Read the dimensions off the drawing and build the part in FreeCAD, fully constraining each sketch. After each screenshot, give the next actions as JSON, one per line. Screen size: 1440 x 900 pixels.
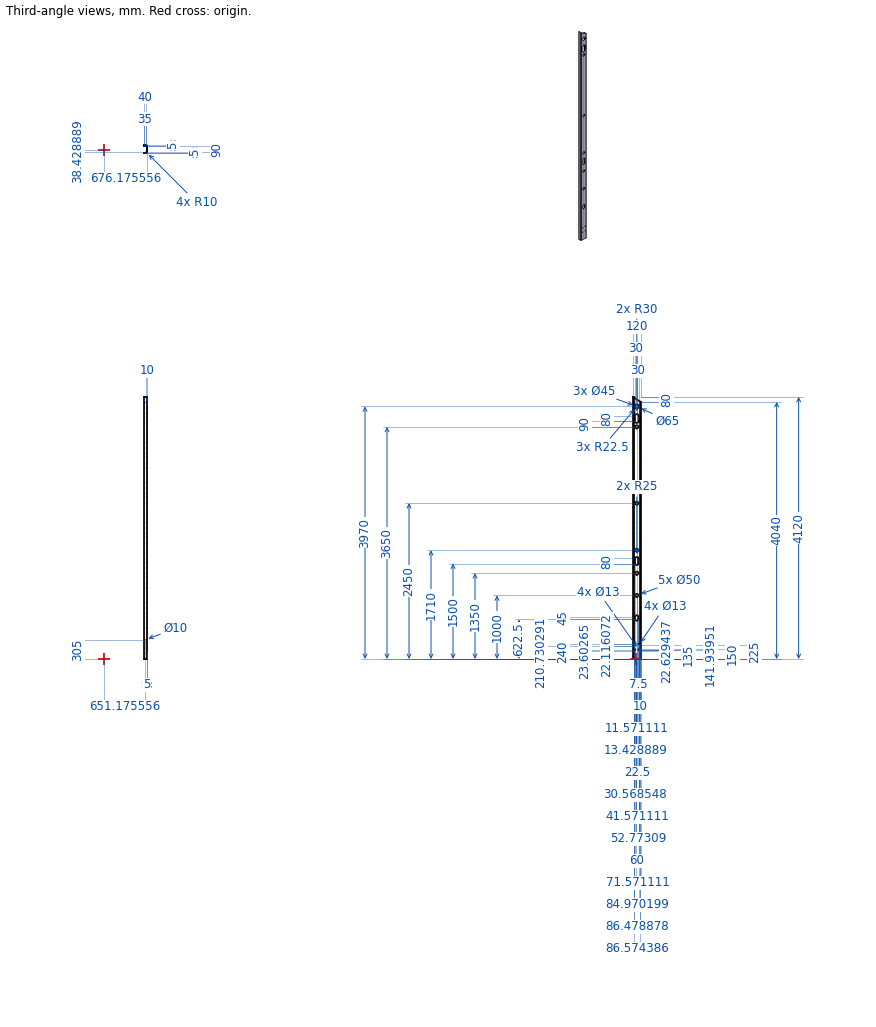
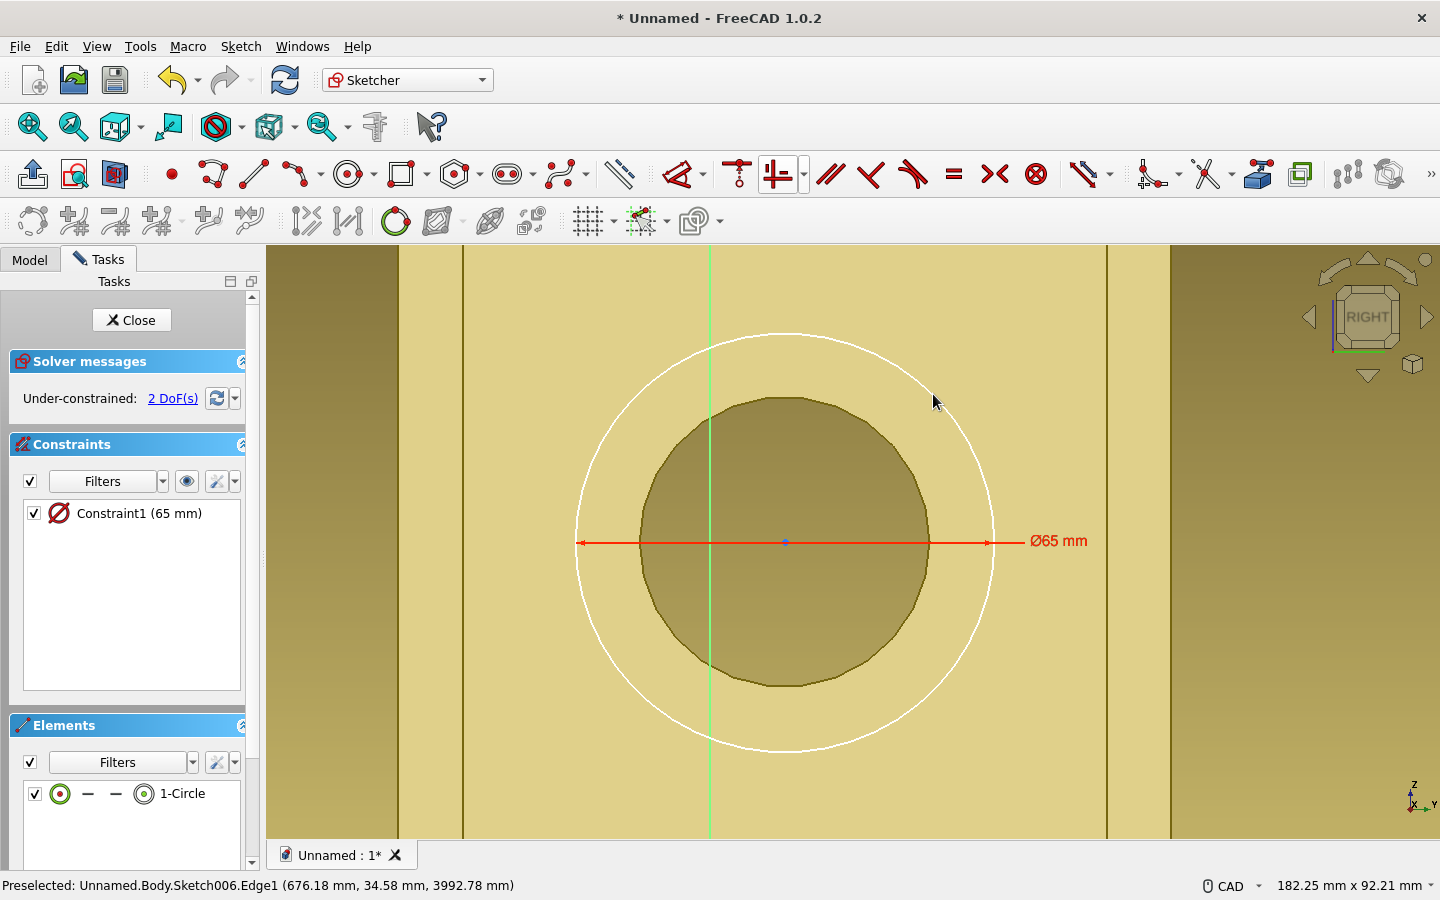
{"action": "key", "text": "d"}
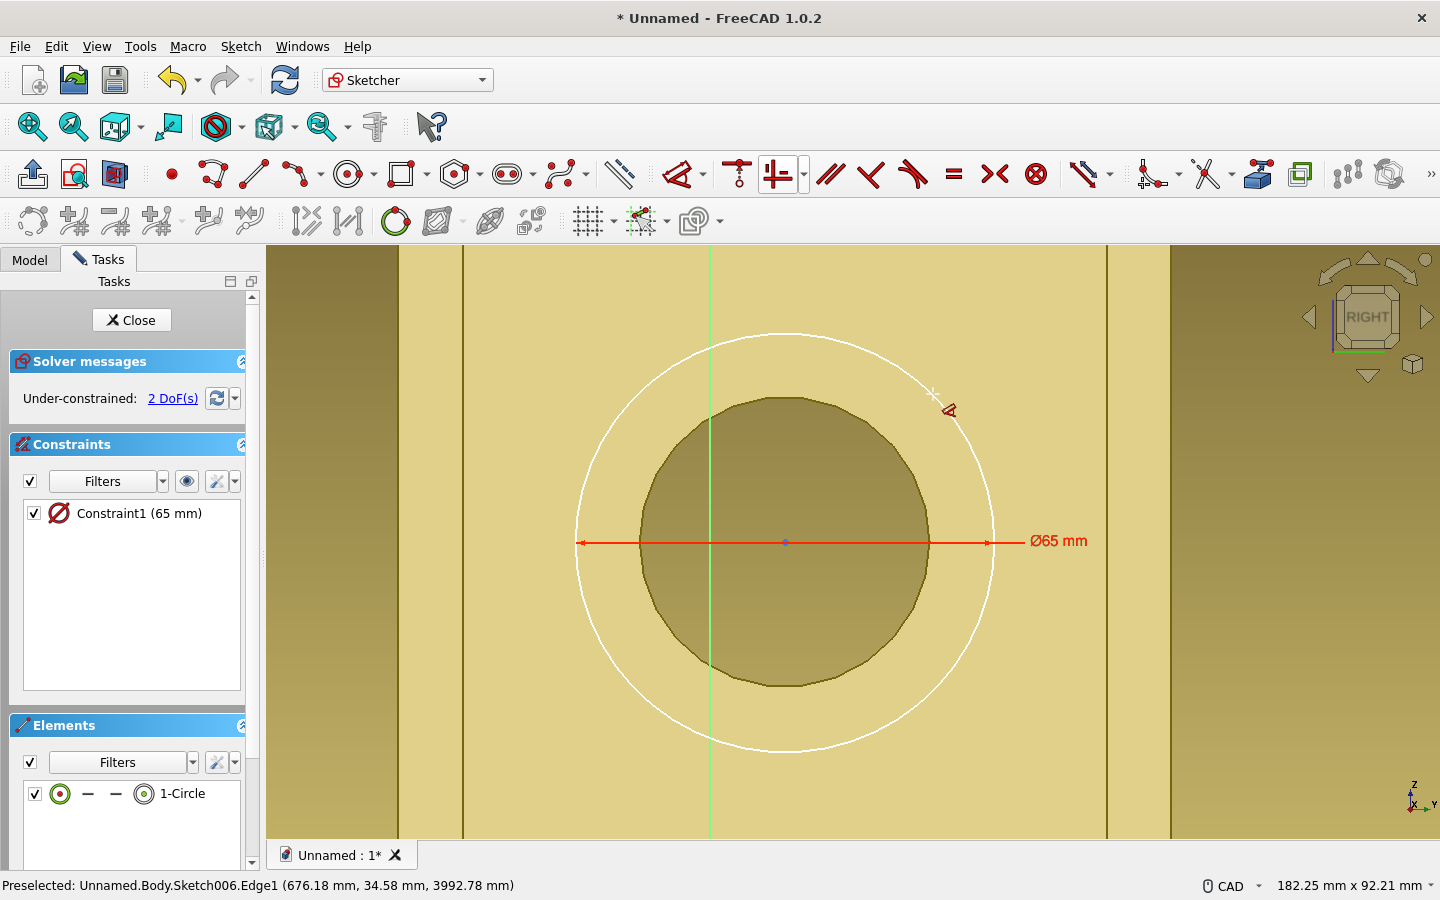
{"action": "left_click", "coordinate": [785, 543]}
{"action": "left_click", "coordinate": [676, 677]}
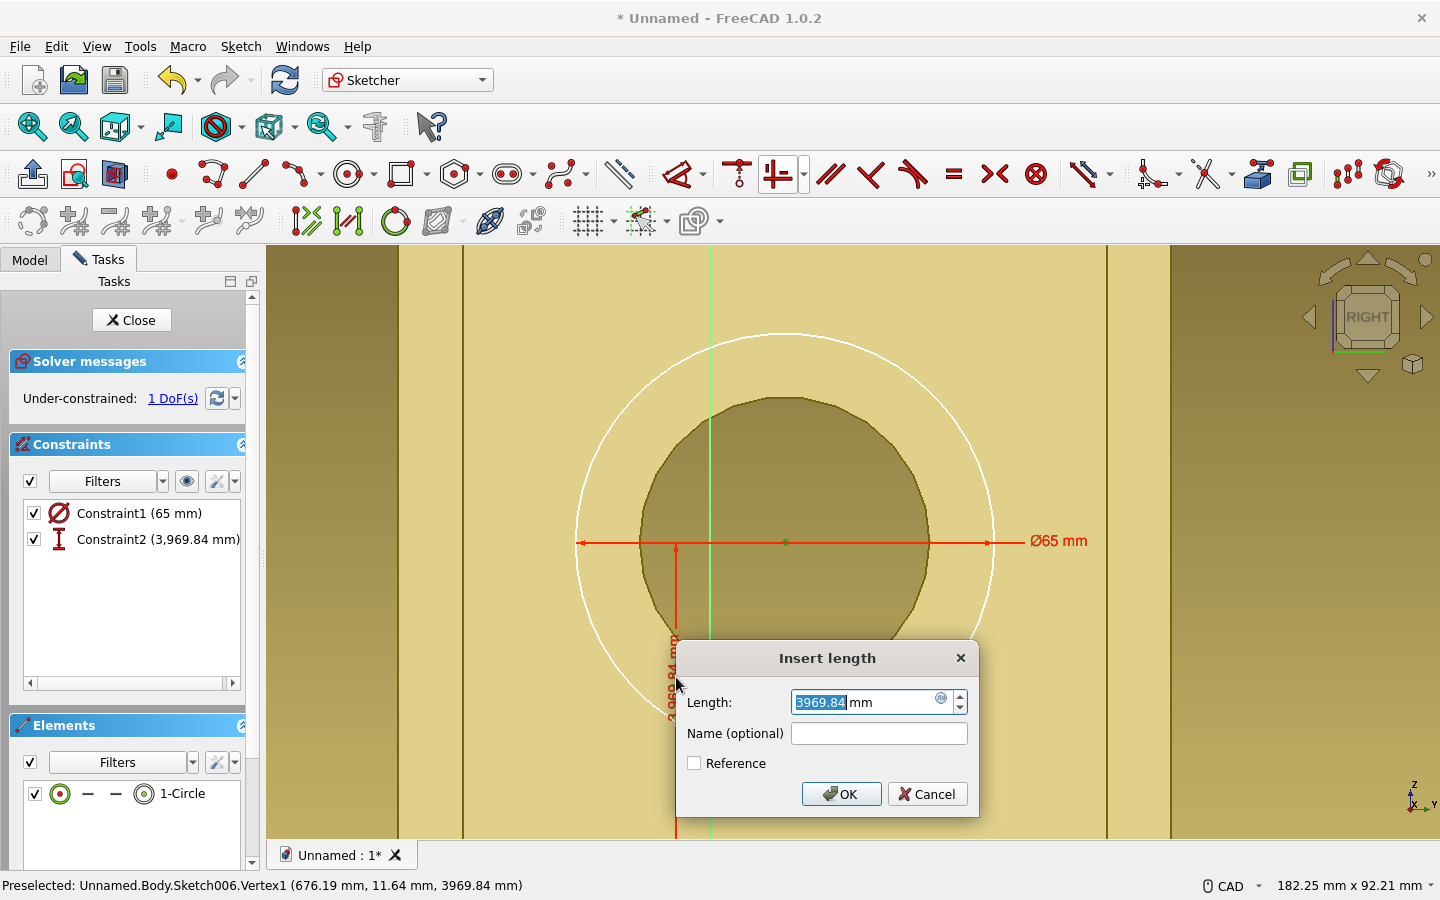
{"action": "type", "text": "3970"}
{"action": "key", "text": "Return"}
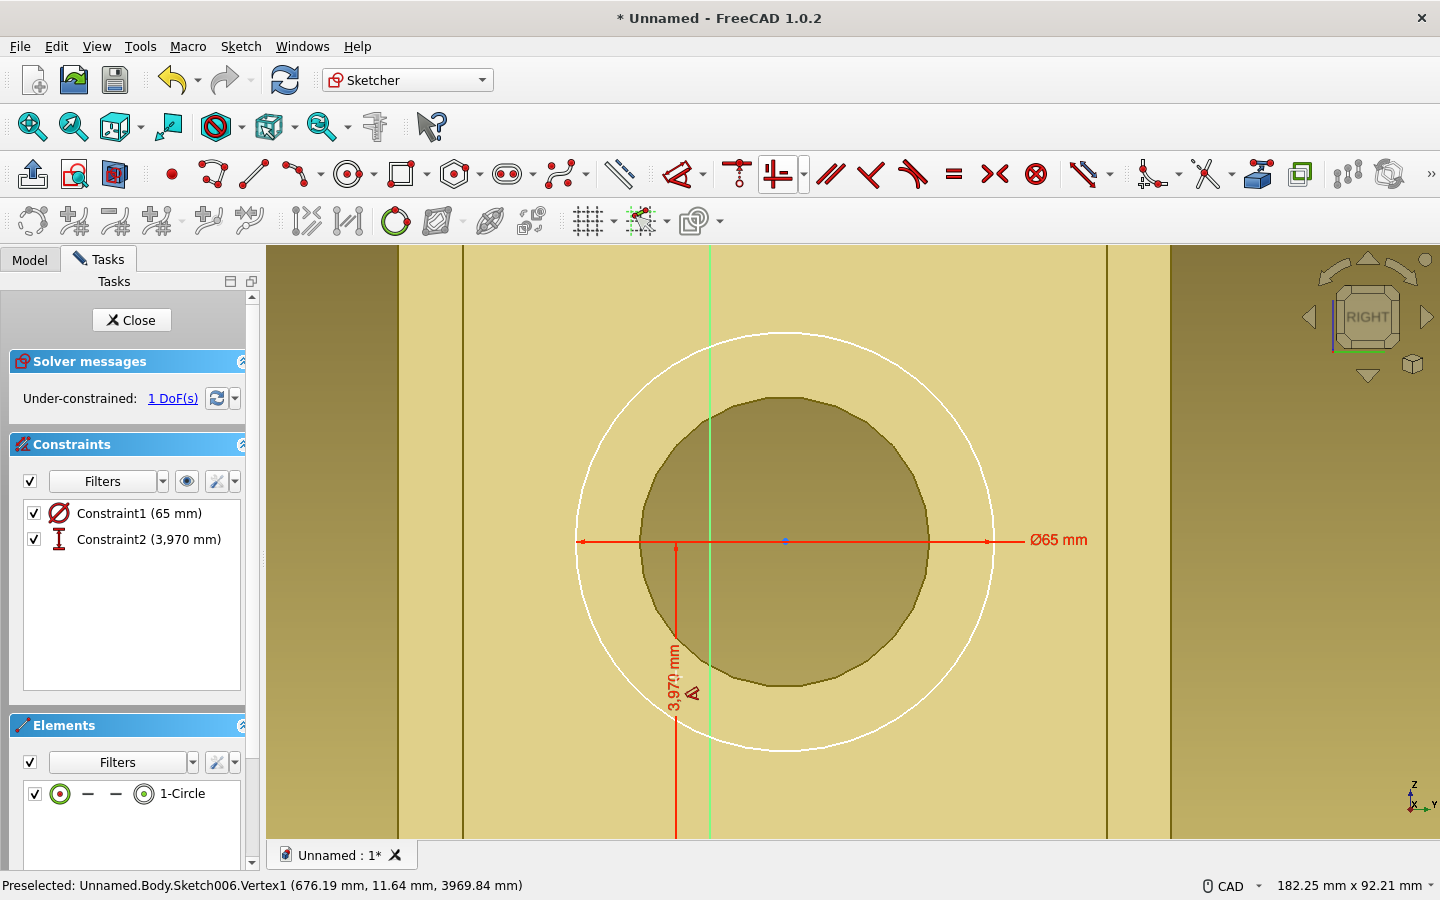
{"action": "left_click", "coordinate": [785, 542]}
{"action": "left_click", "coordinate": [748, 508]}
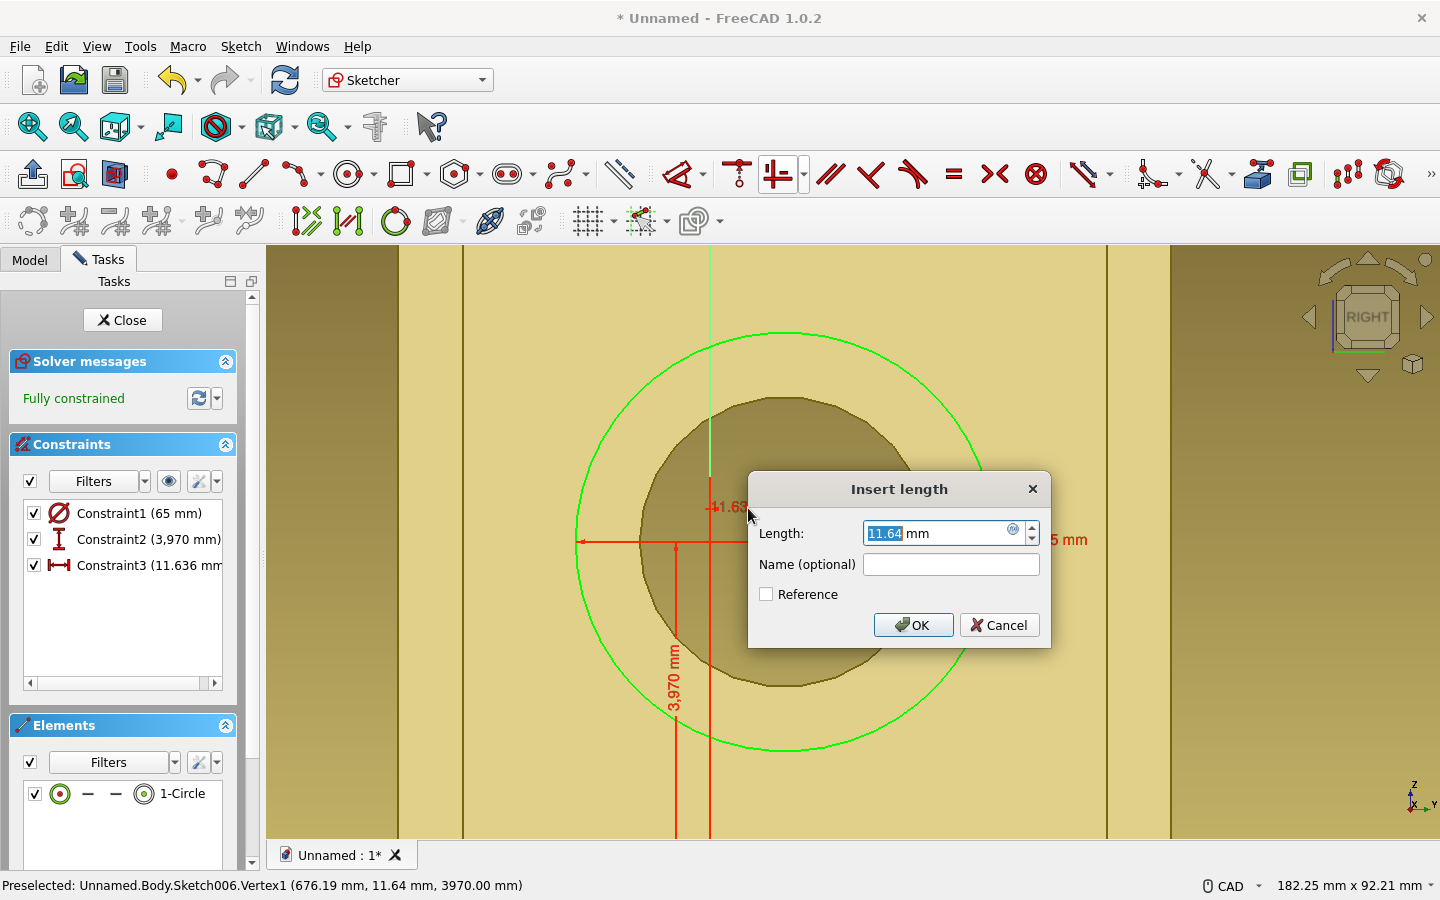
{"action": "type", "text": "11.571111"}
{"action": "key", "text": "Return"}
{"action": "key", "text": "Escape"}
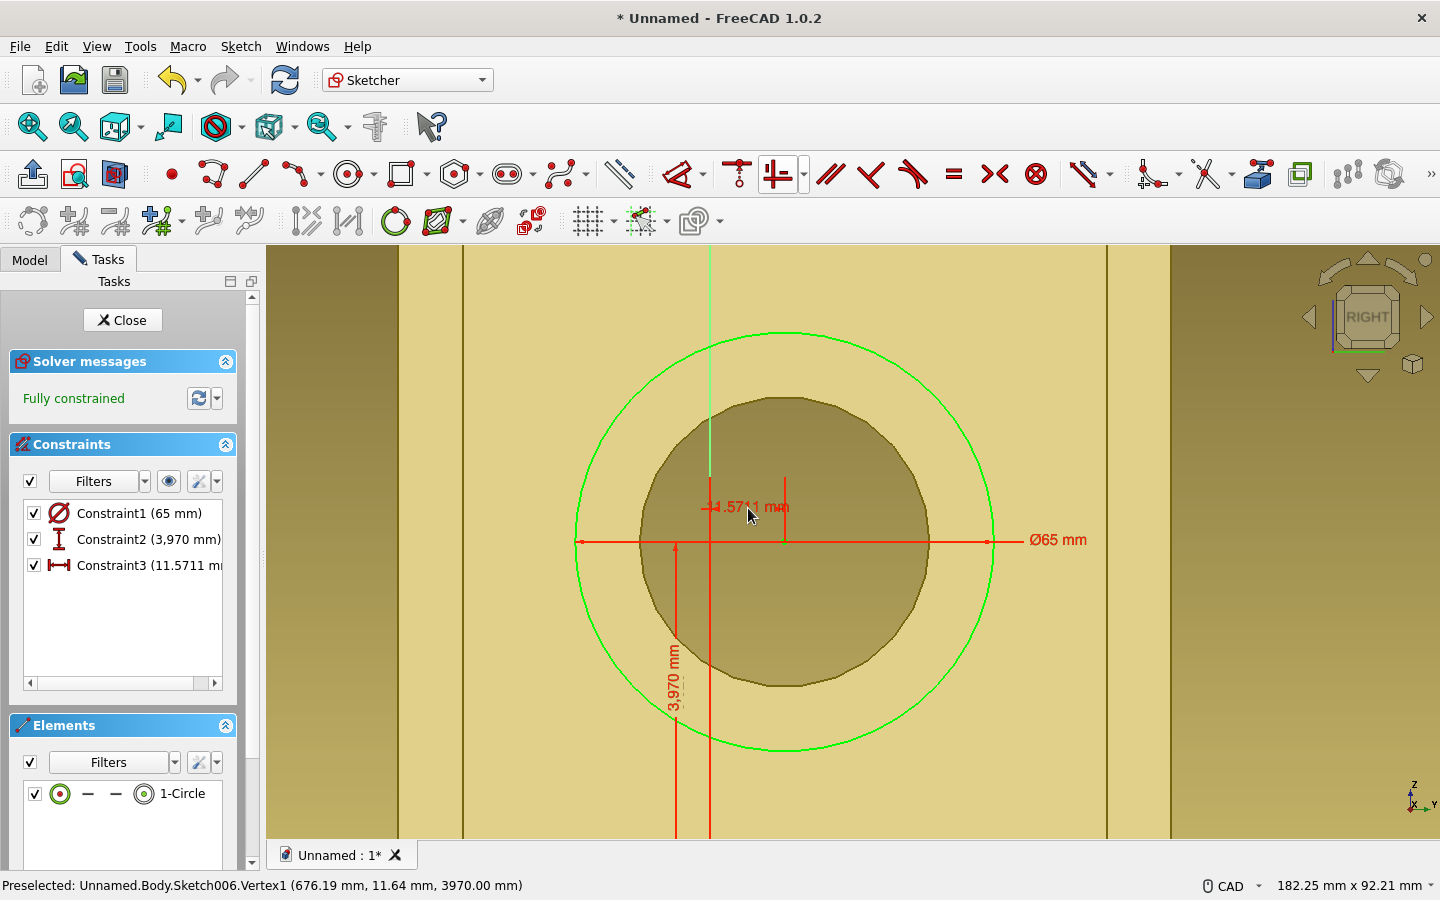
{"action": "left_click", "coordinate": [123, 320]}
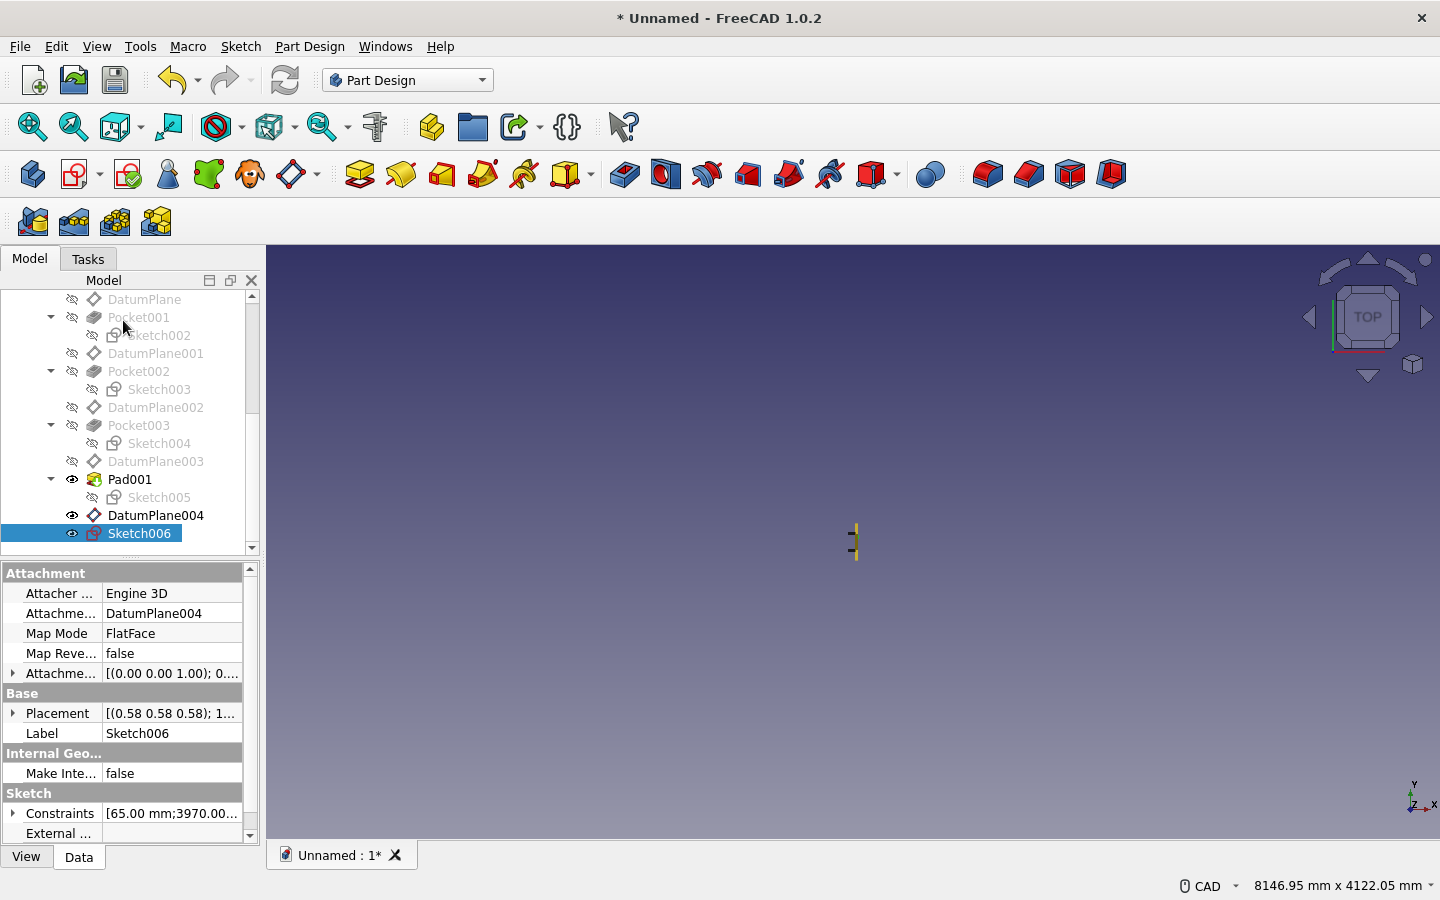
{"action": "left_click", "coordinate": [625, 174]}